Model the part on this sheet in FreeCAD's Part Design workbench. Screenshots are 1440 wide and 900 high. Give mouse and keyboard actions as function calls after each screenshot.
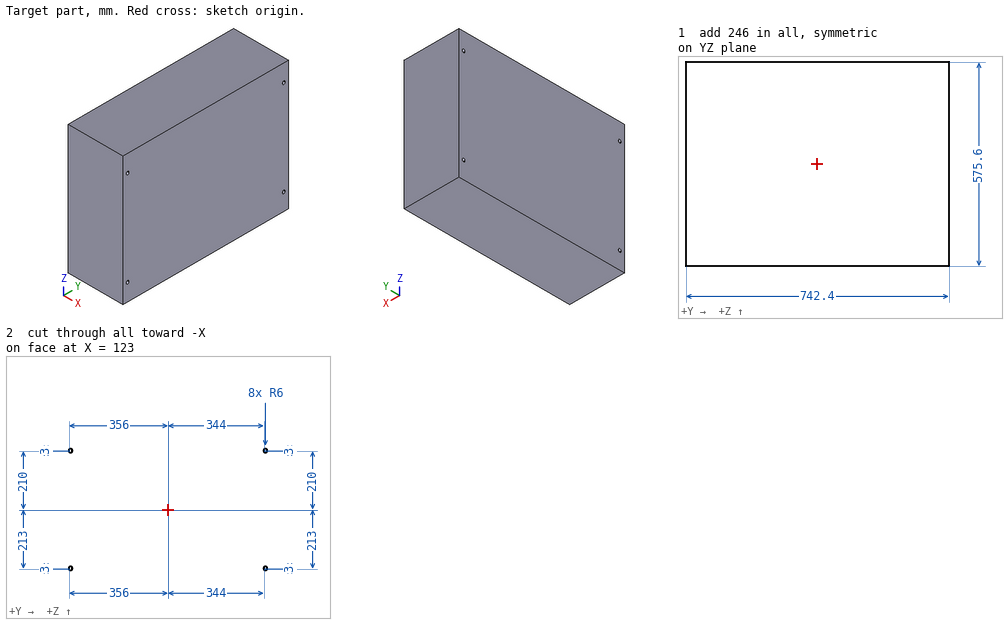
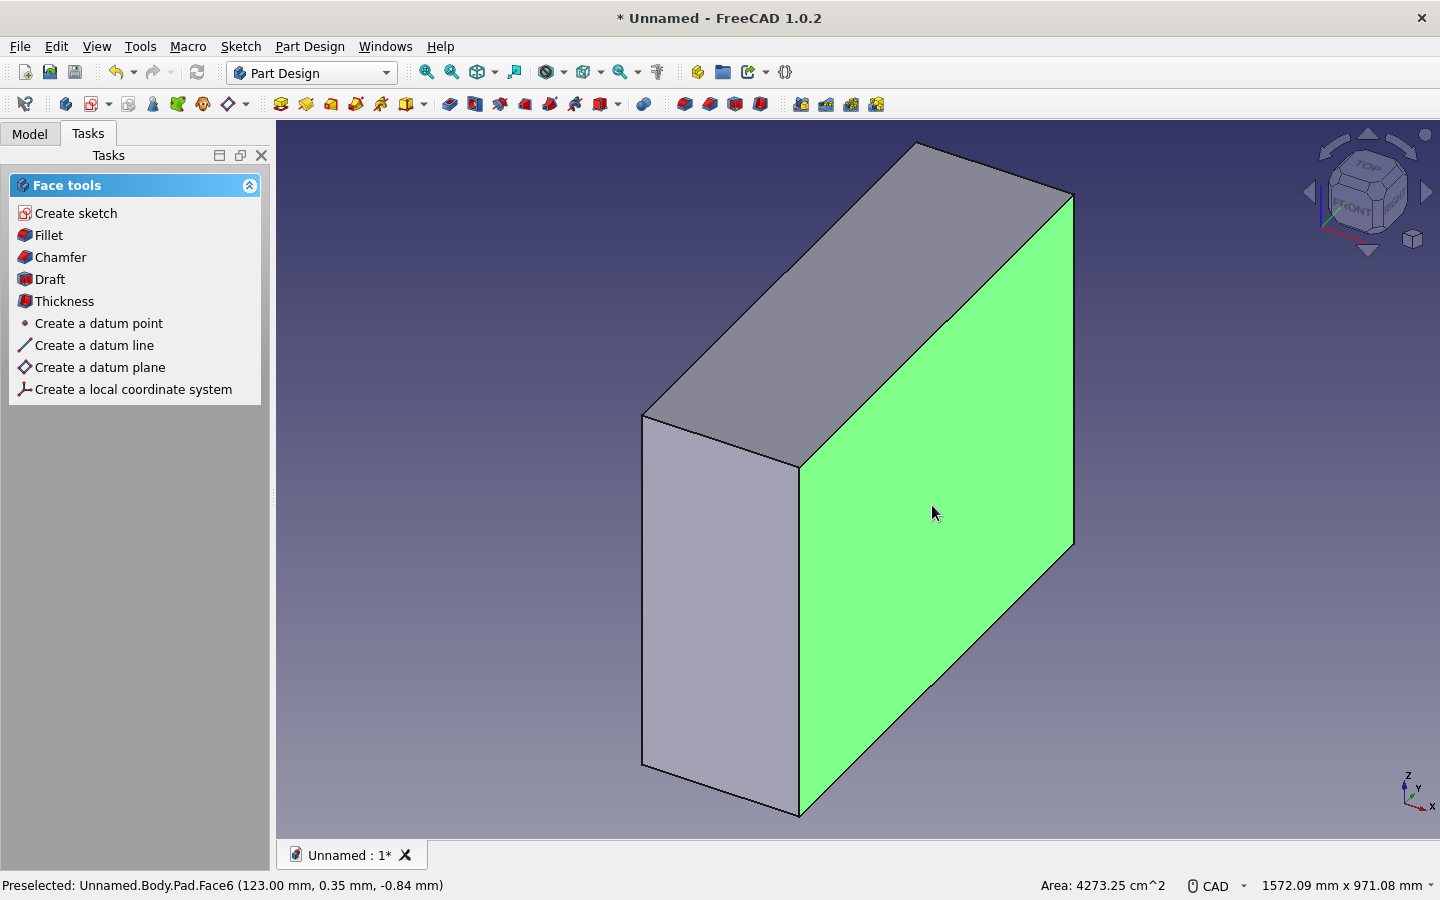
click(90, 104)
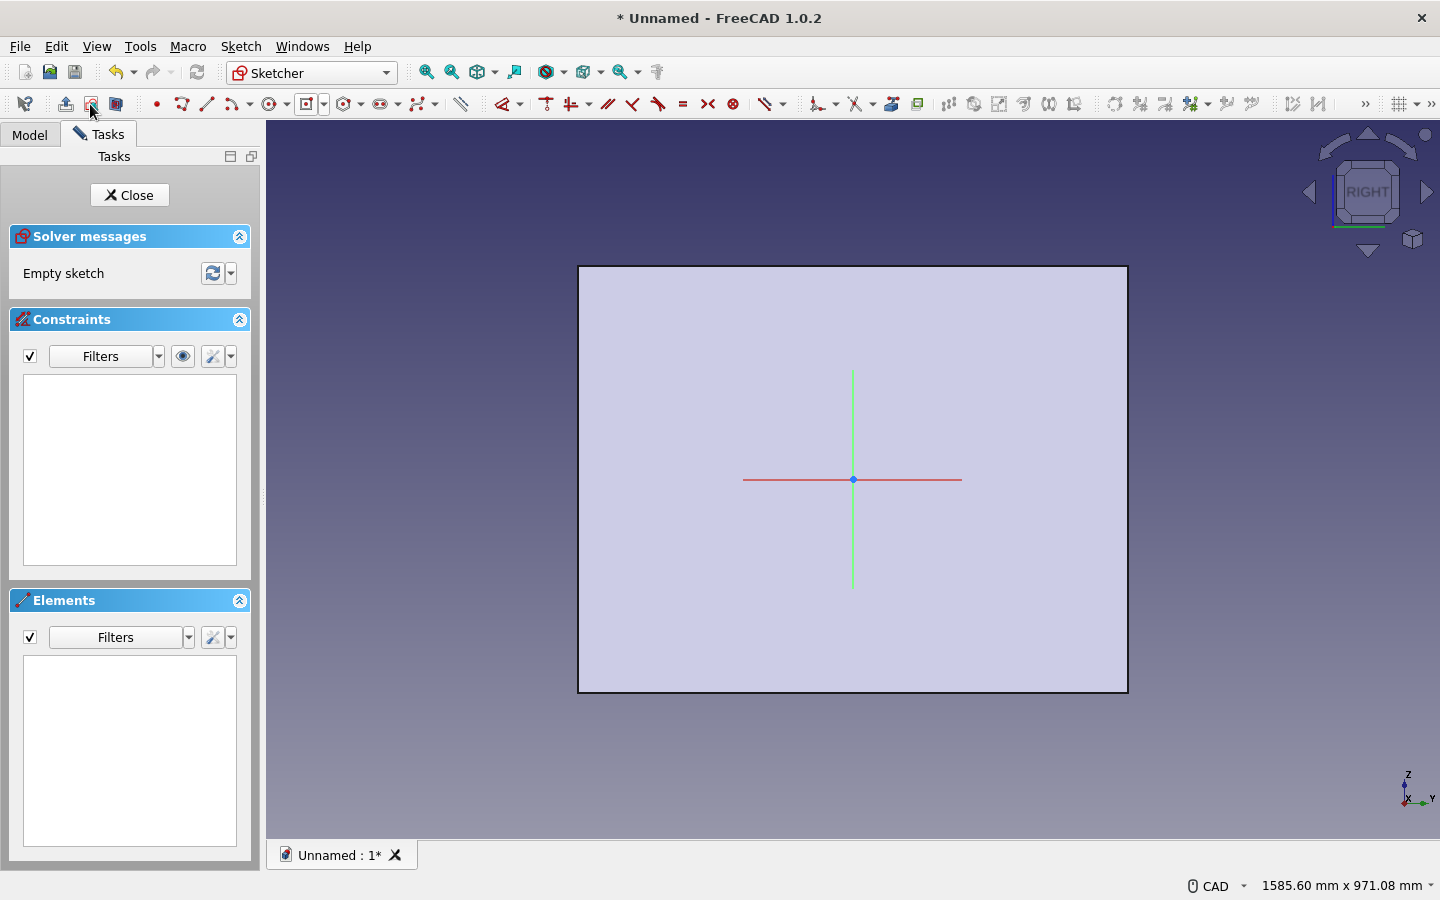
click(380, 104)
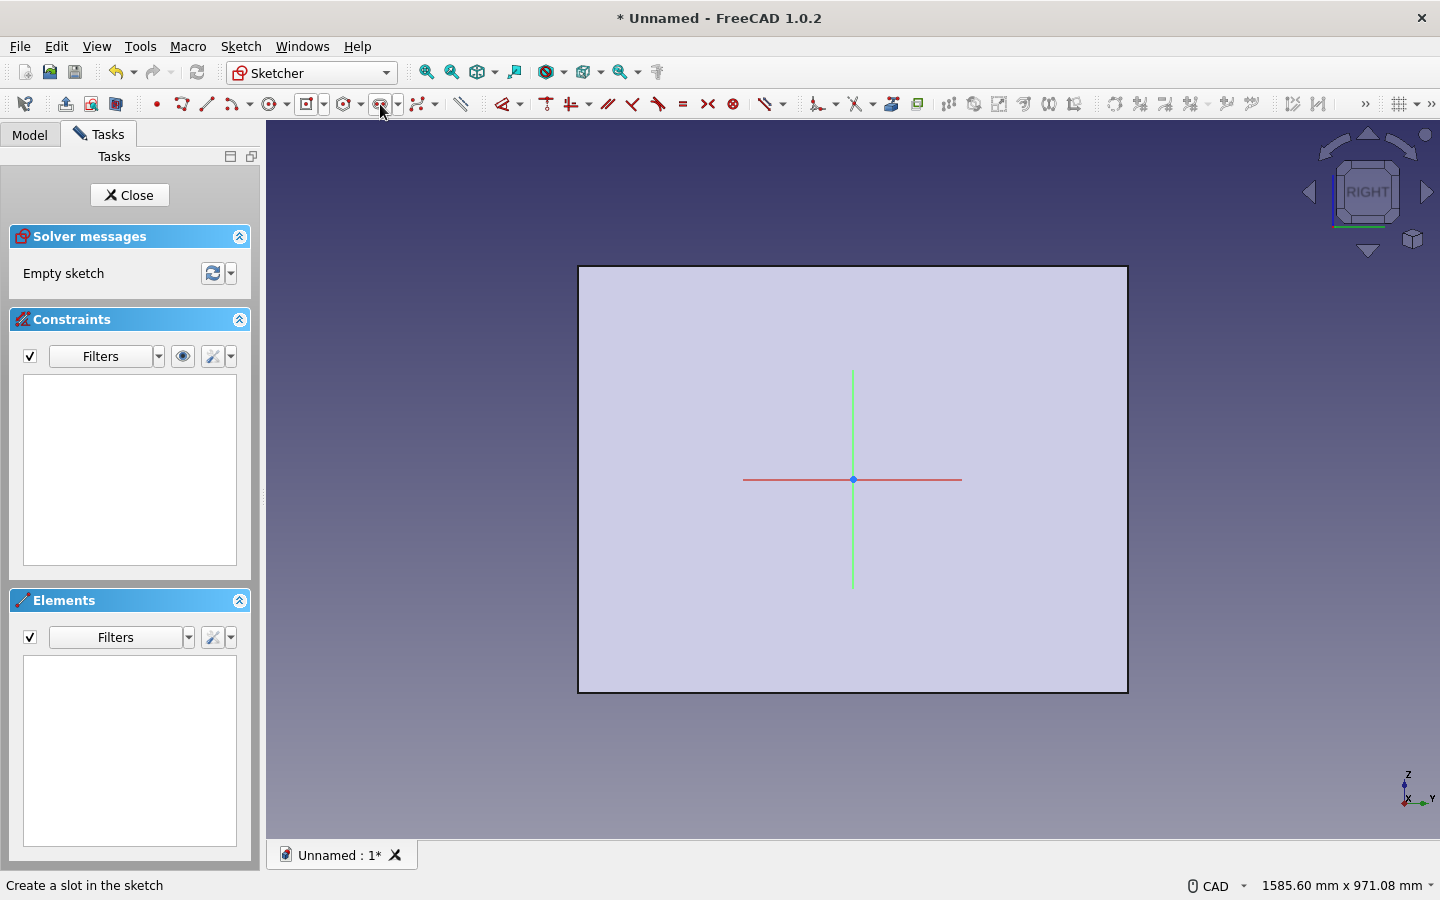
scroll(1112, 324, up, 9)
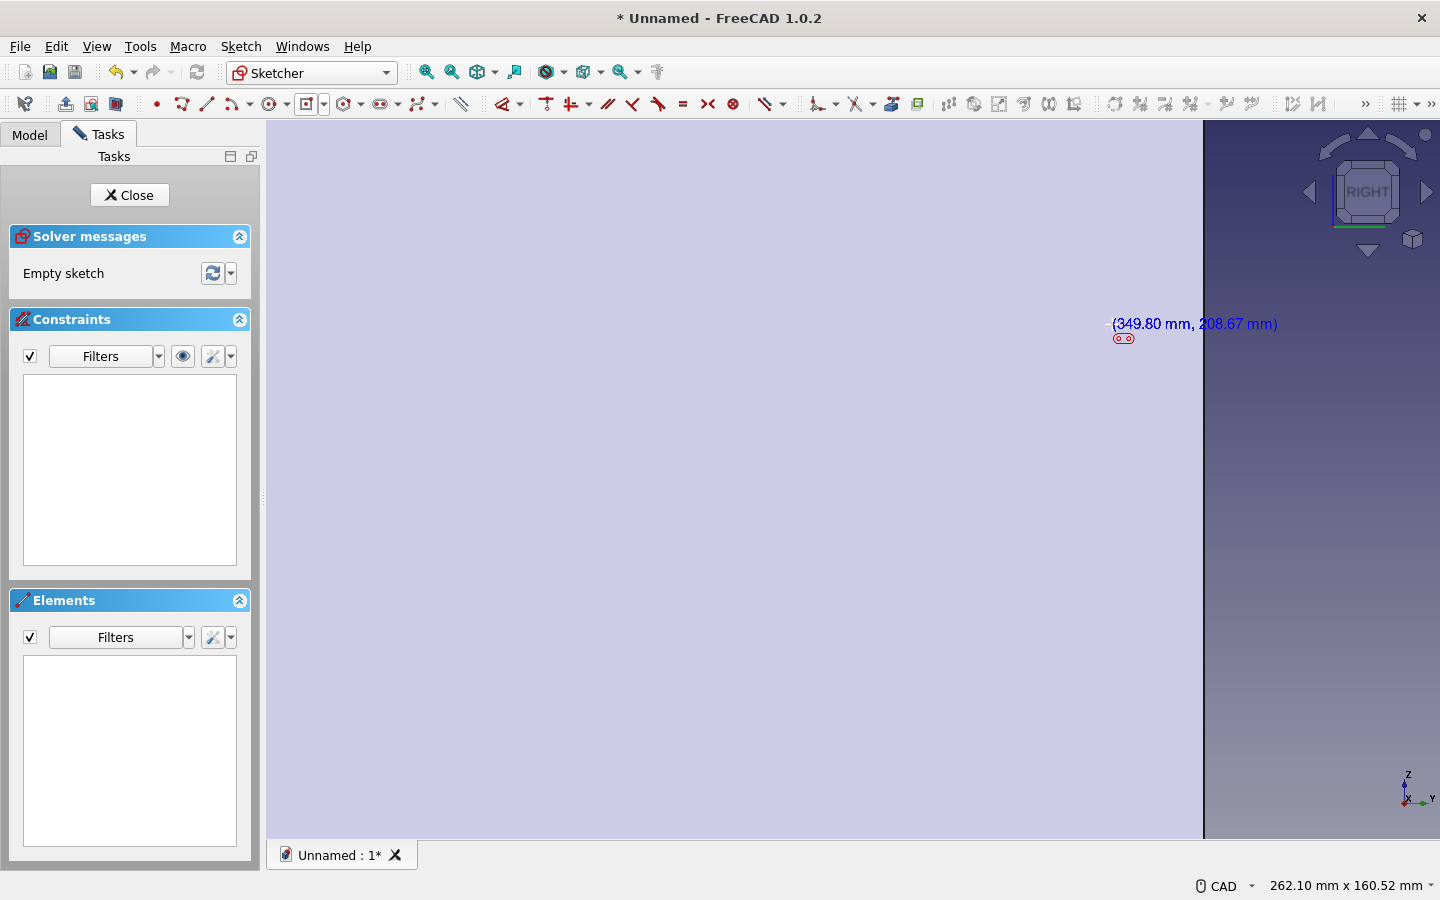
scroll(1099, 281, down, 8)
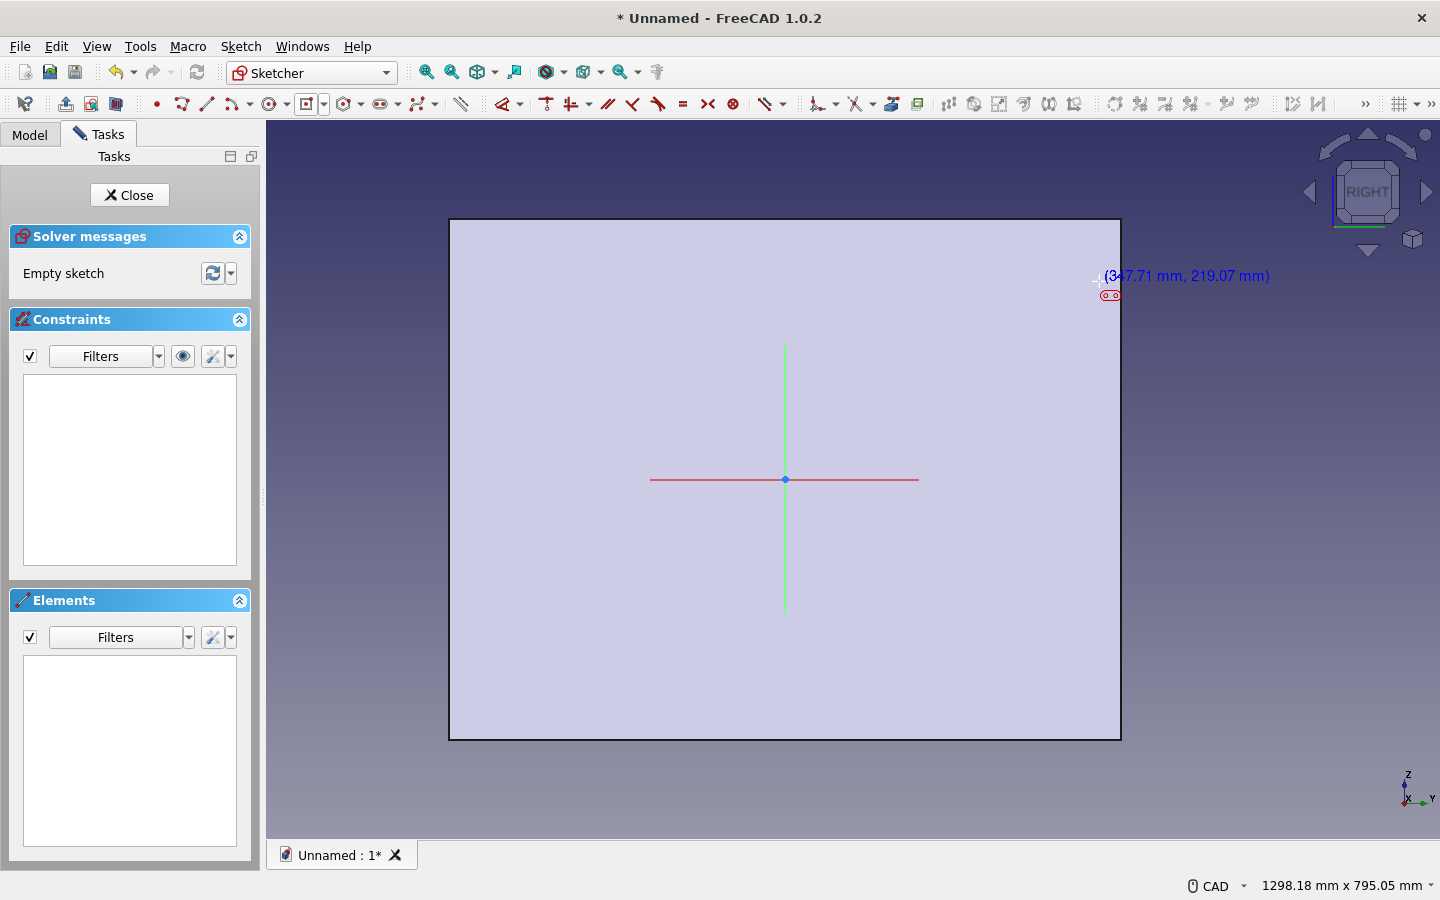
click(1102, 290)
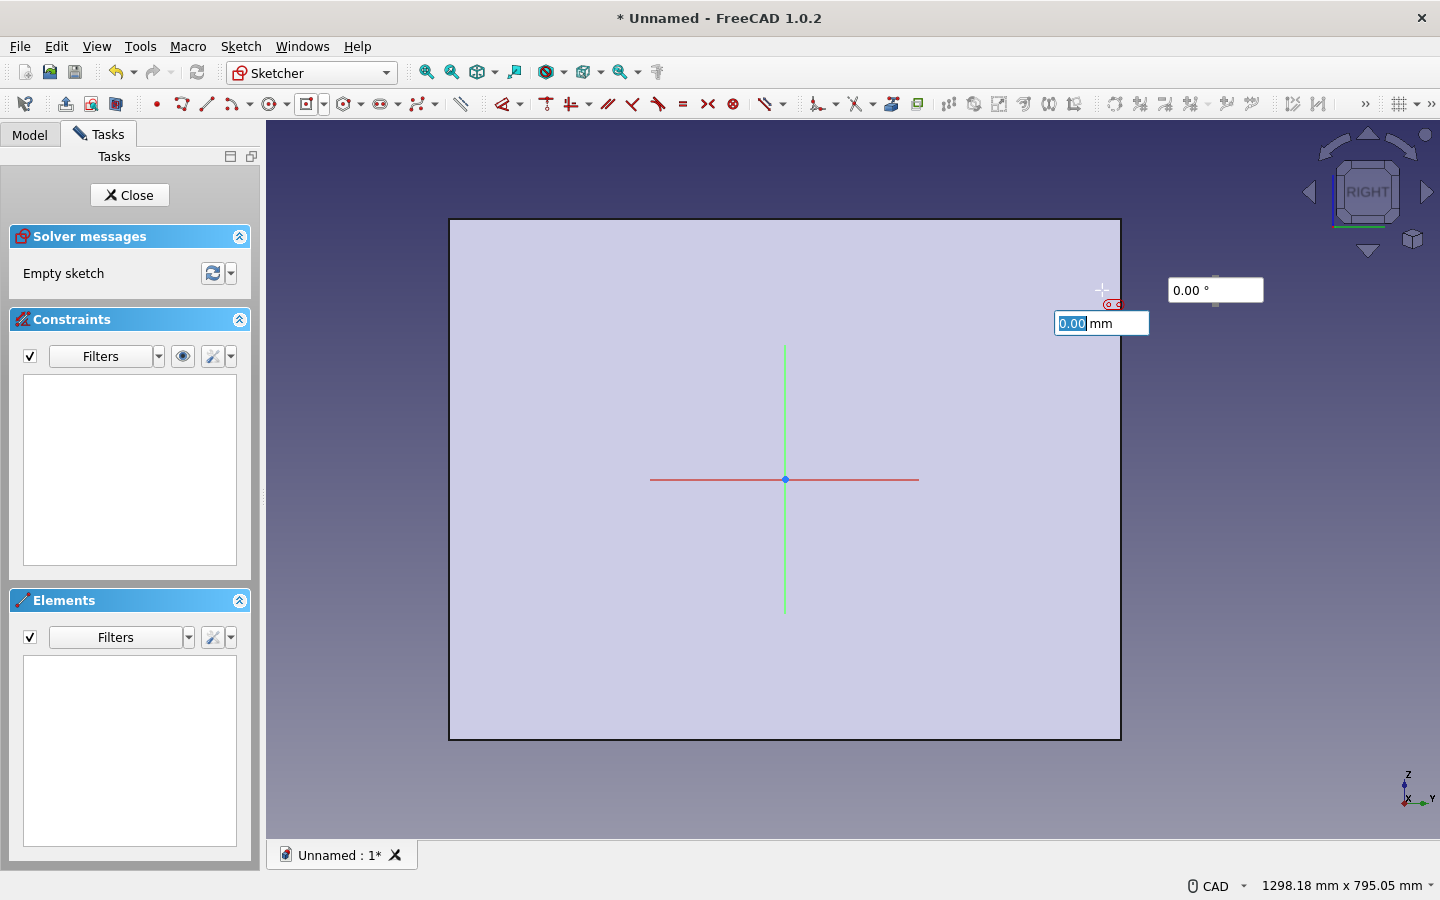
scroll(1102, 287, up, 9)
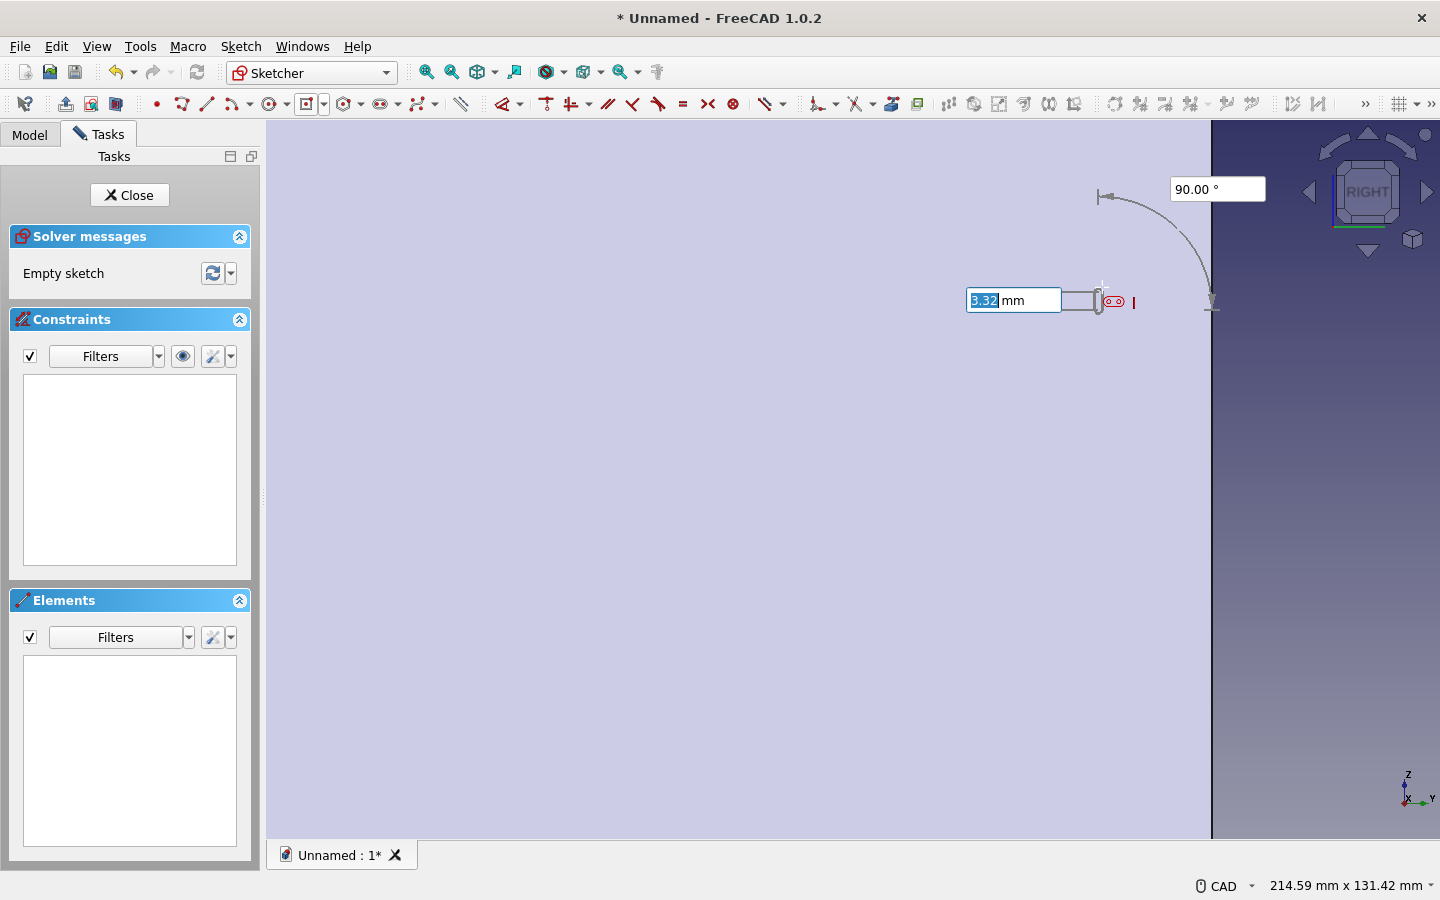
click(1098, 285)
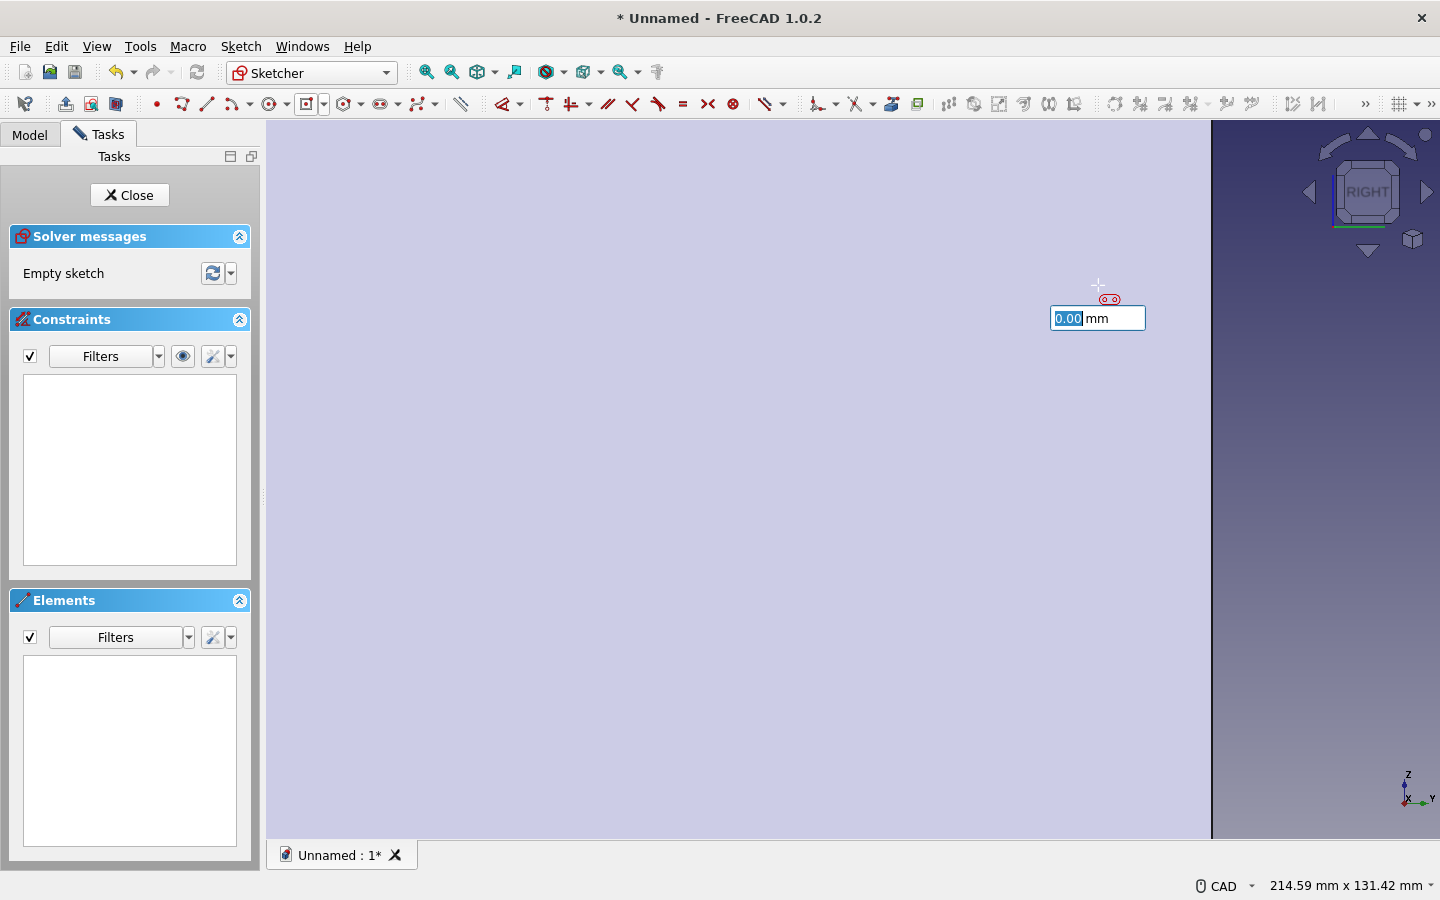
click(1129, 293)